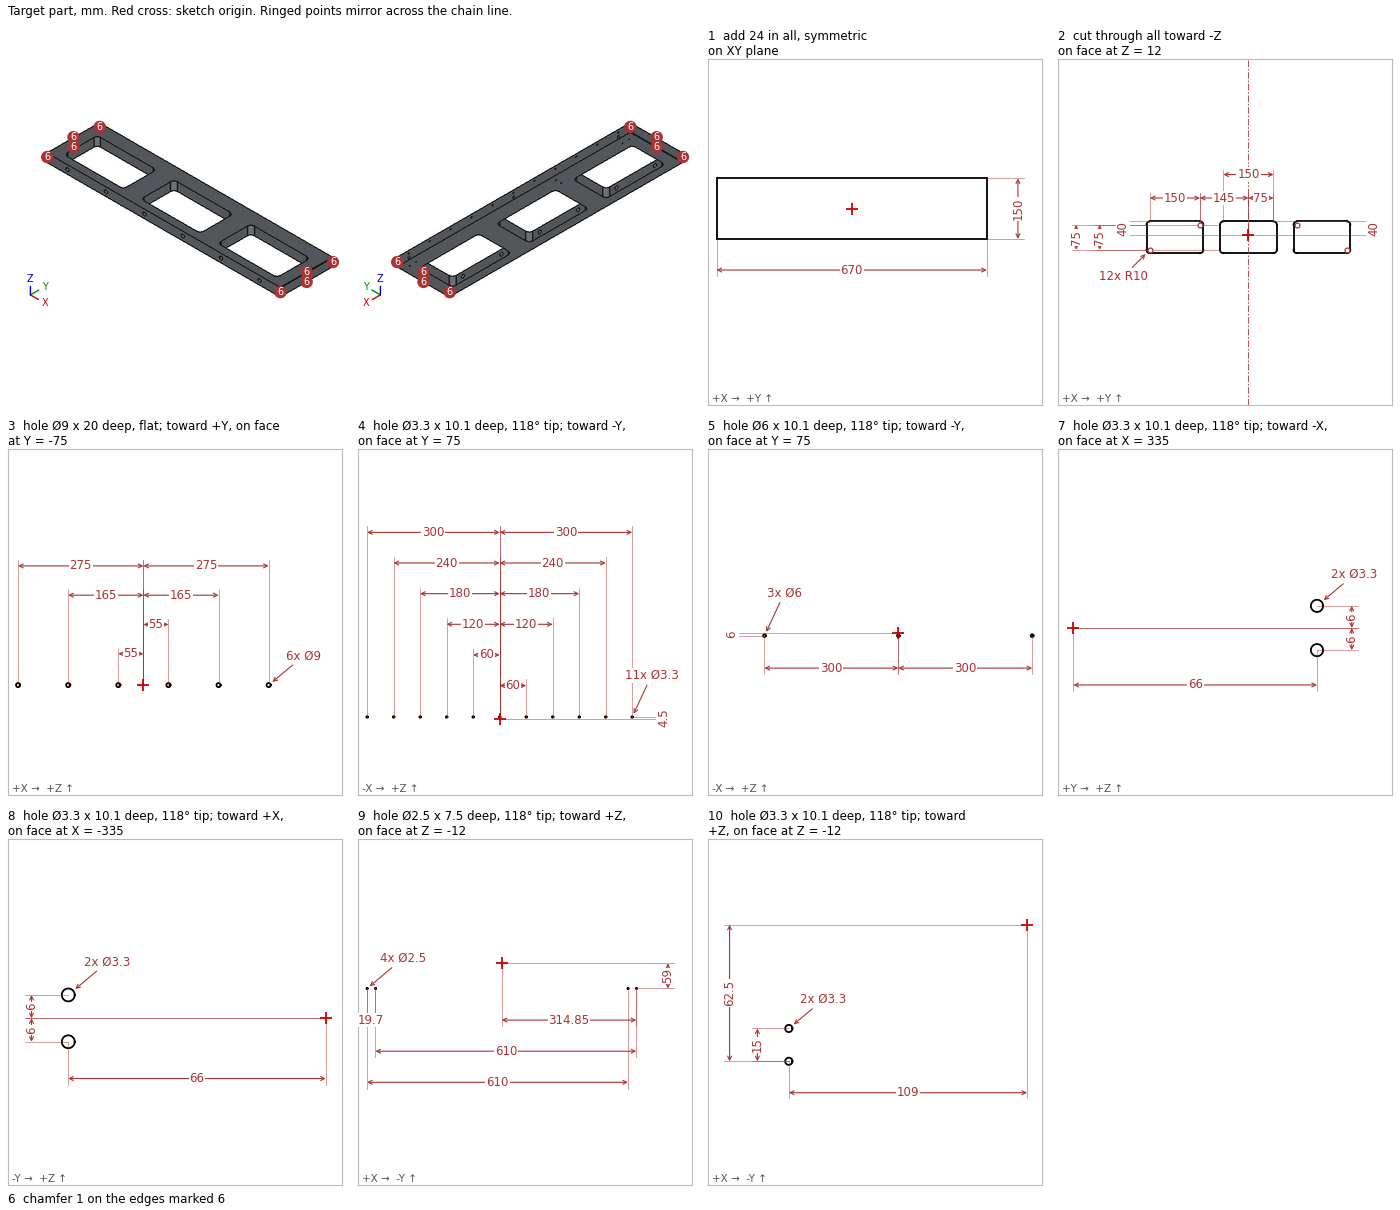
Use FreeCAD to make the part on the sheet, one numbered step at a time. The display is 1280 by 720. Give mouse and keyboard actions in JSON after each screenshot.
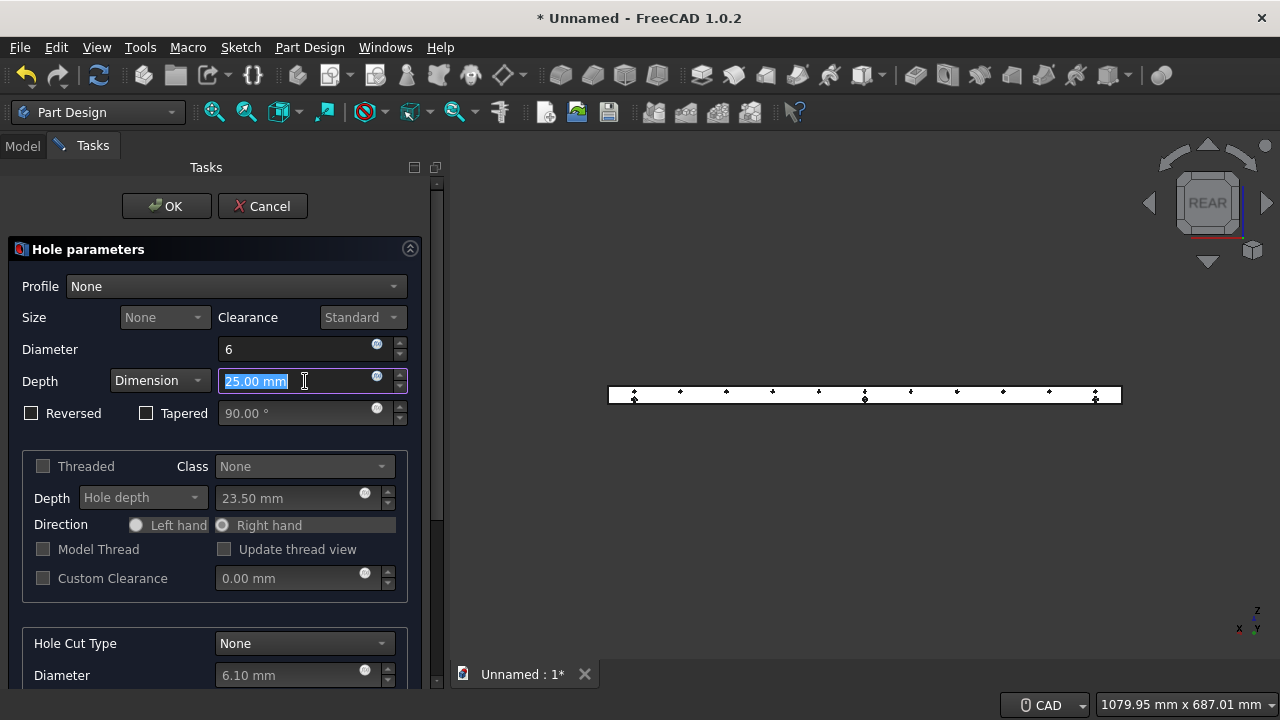
{"action": "type", "text": "10.1"}
{"action": "key", "text": "Tab"}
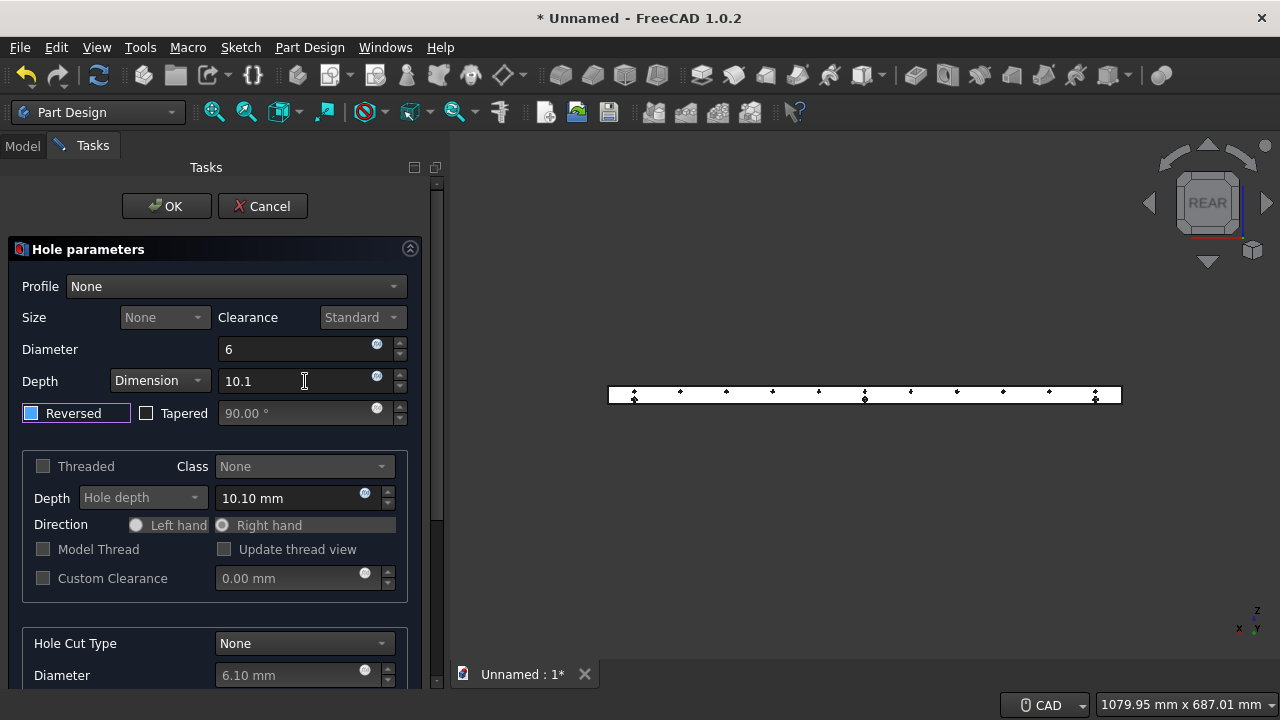
{"action": "left_click", "coordinate": [167, 206]}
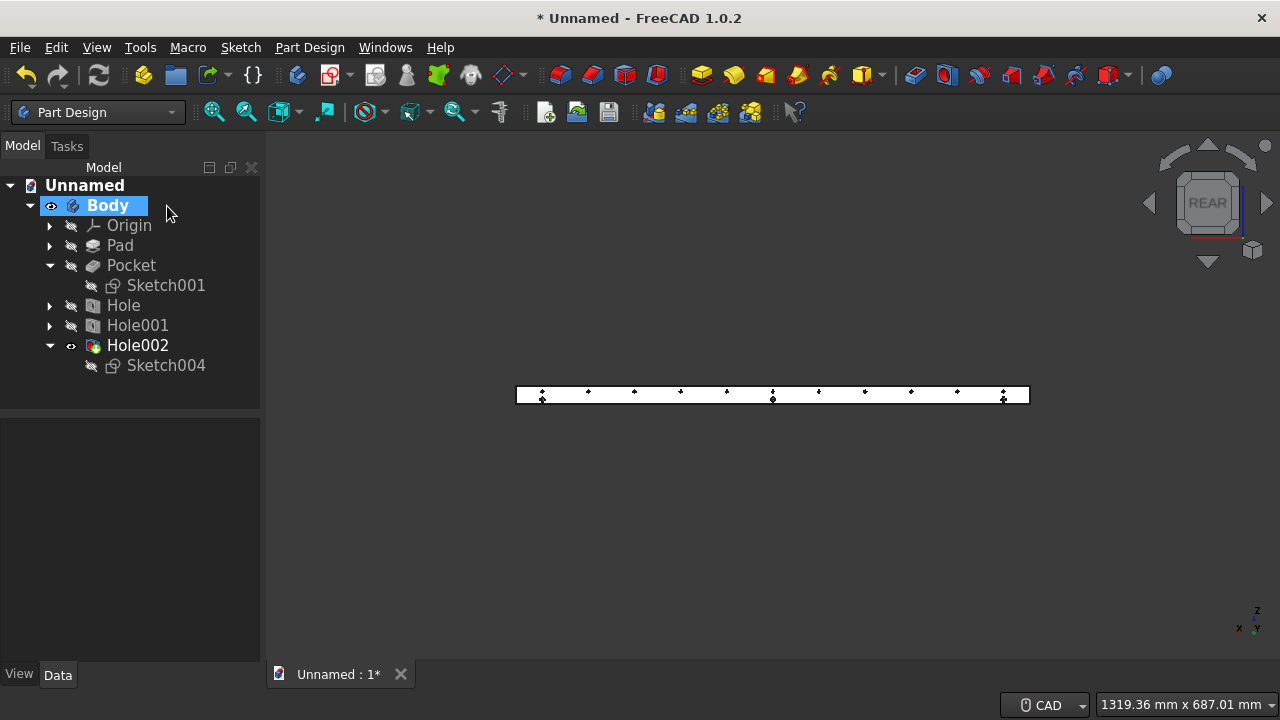
{"action": "key", "text": "0"}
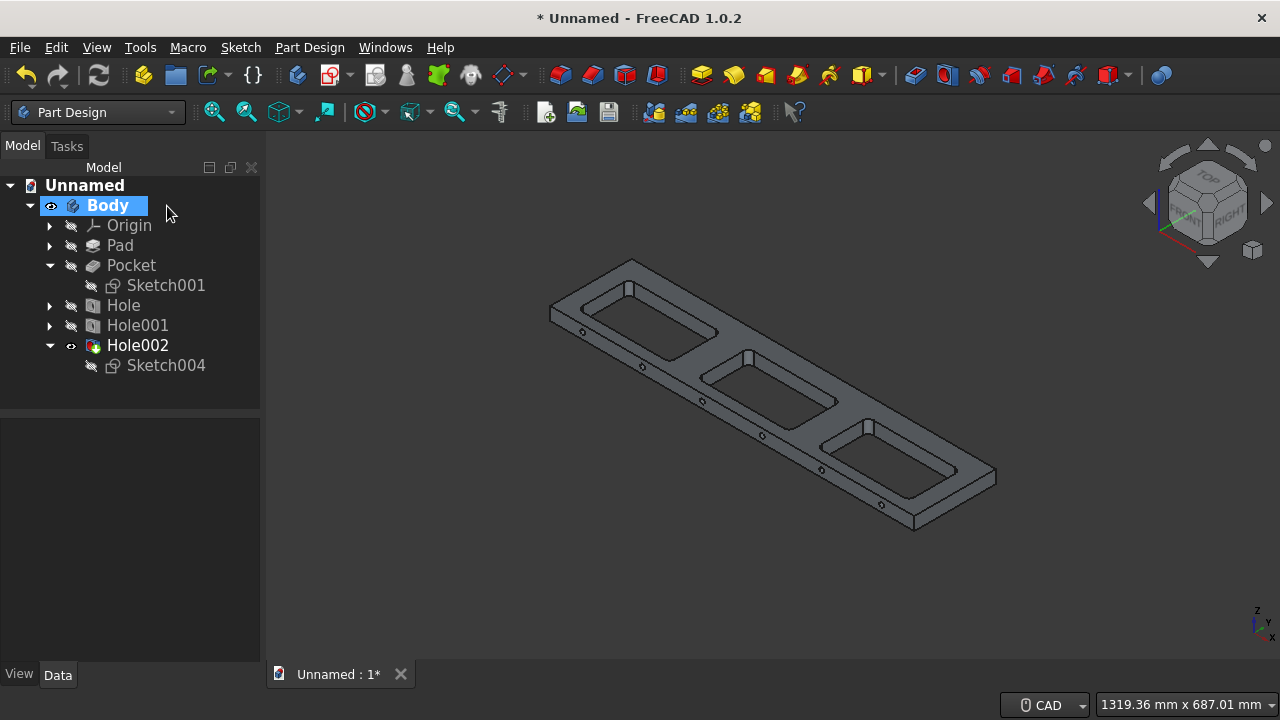
{"action": "key", "text": "2"}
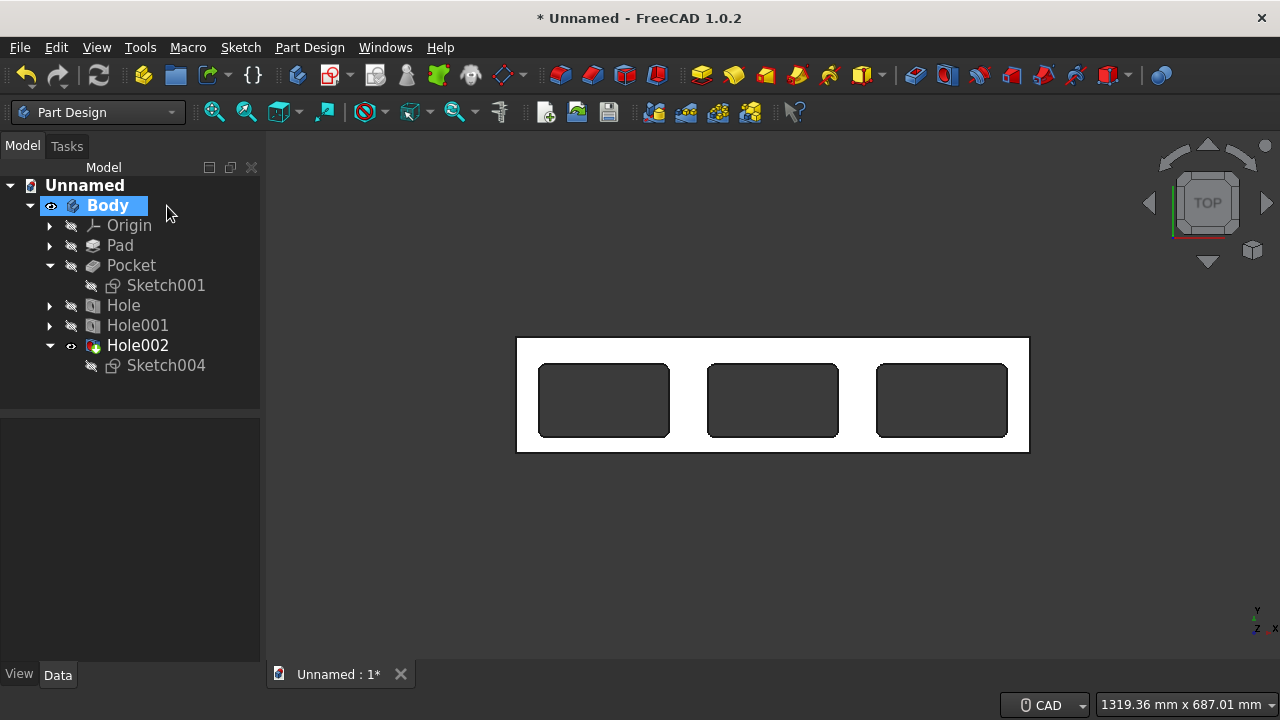
{"action": "key", "text": "1"}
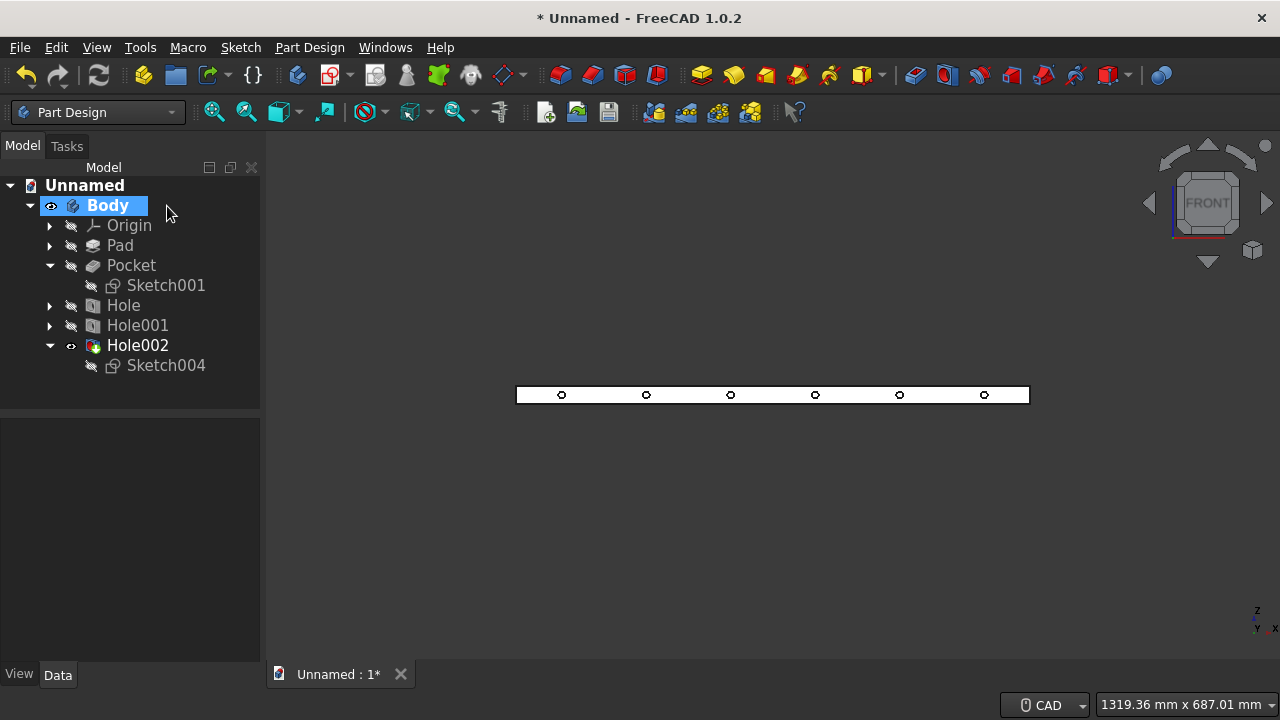
{"action": "key", "text": "3"}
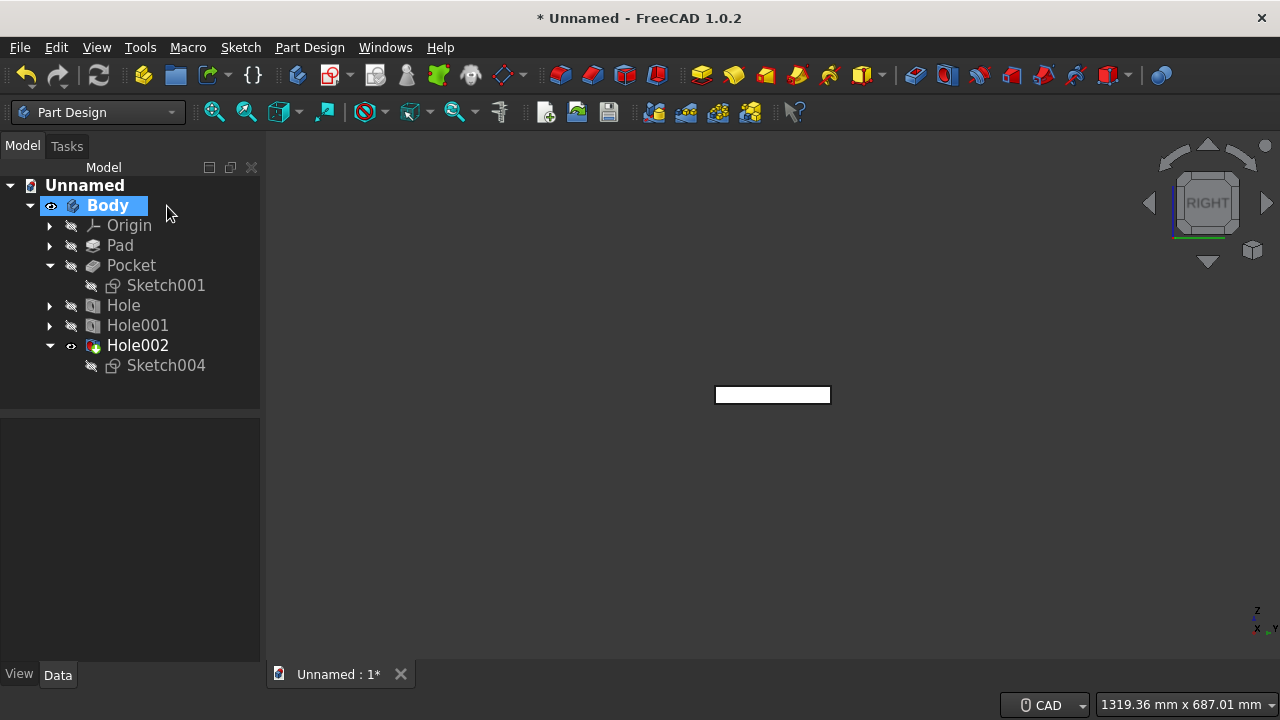
{"action": "left_click", "coordinate": [216, 112]}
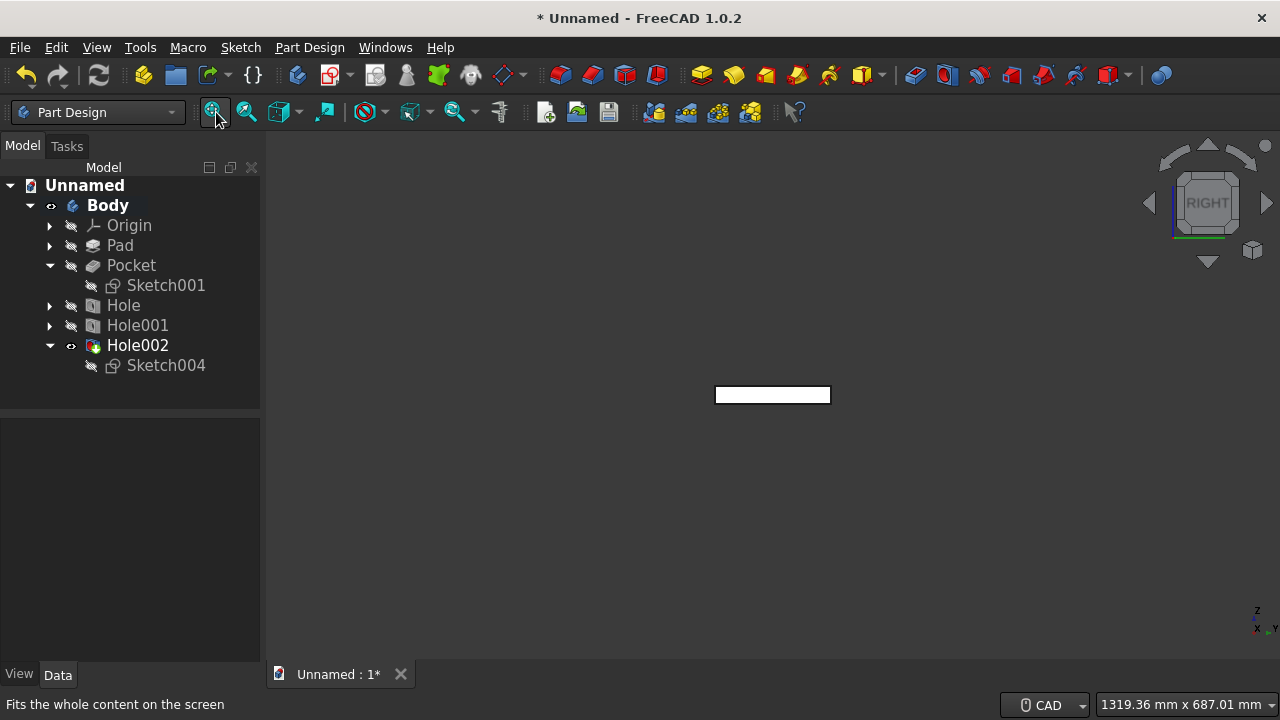
{"action": "left_click", "coordinate": [806, 394]}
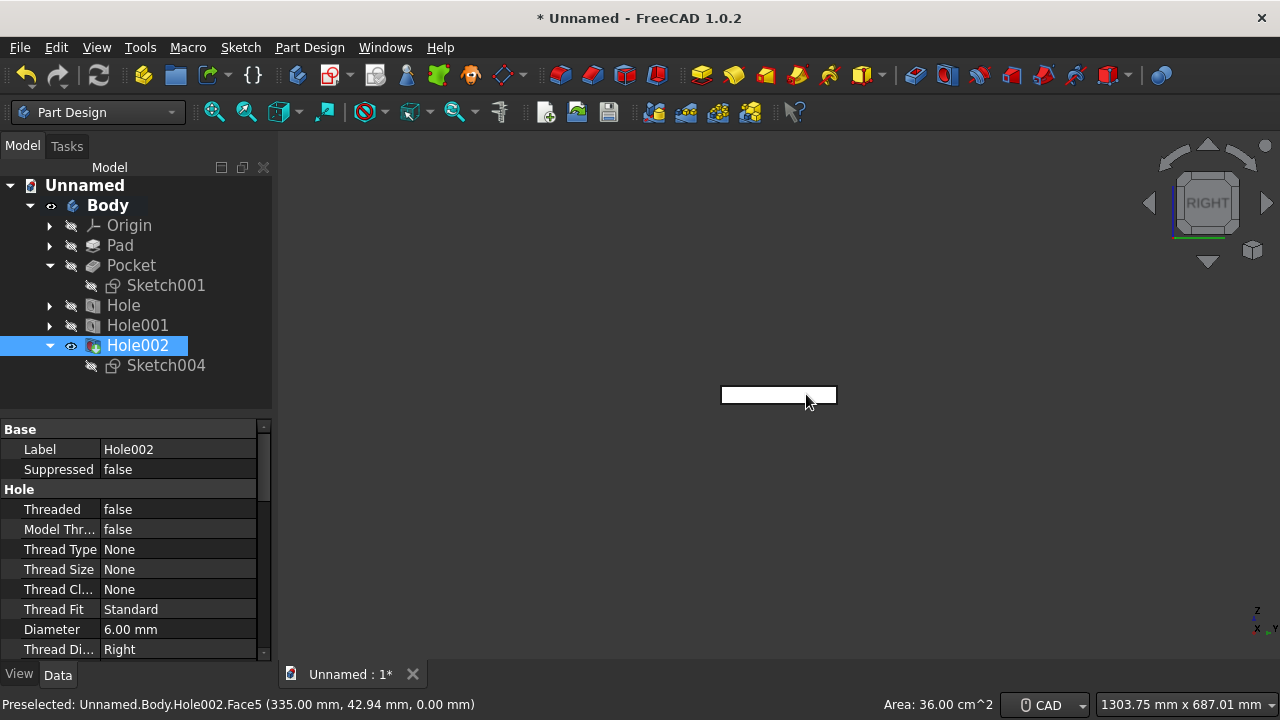
{"action": "key", "text": "5"}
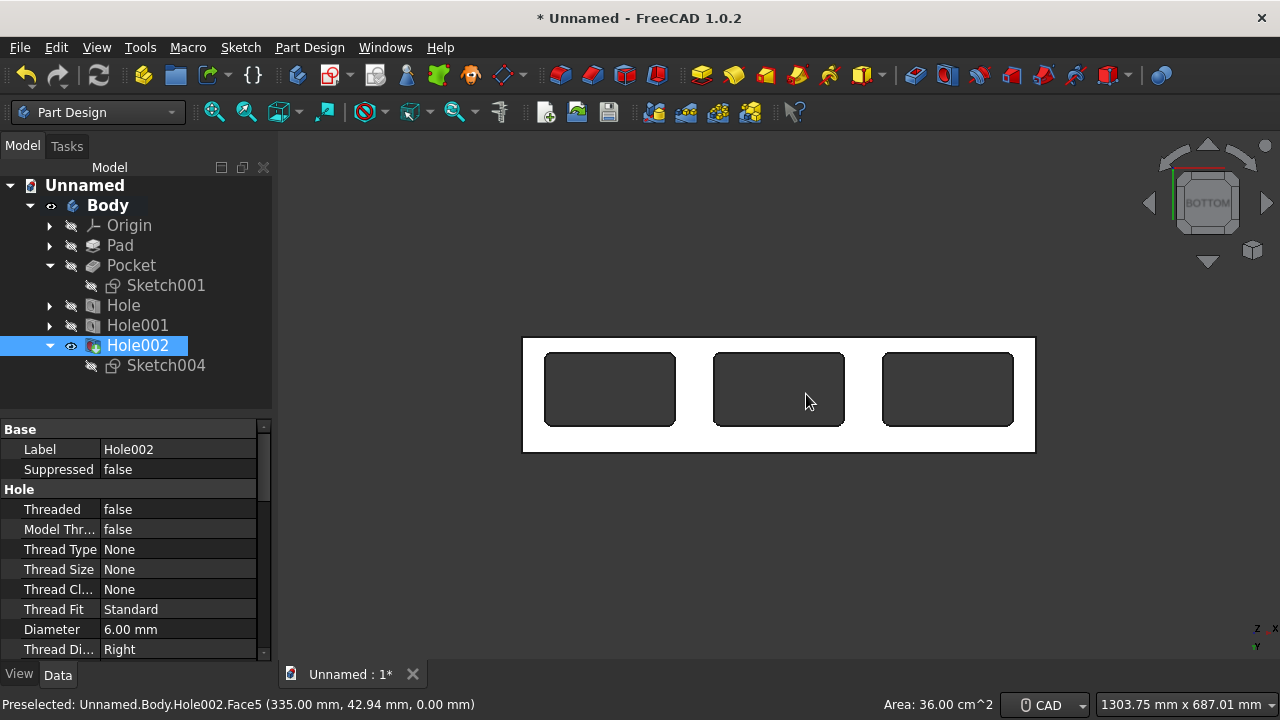
{"action": "key", "text": "4"}